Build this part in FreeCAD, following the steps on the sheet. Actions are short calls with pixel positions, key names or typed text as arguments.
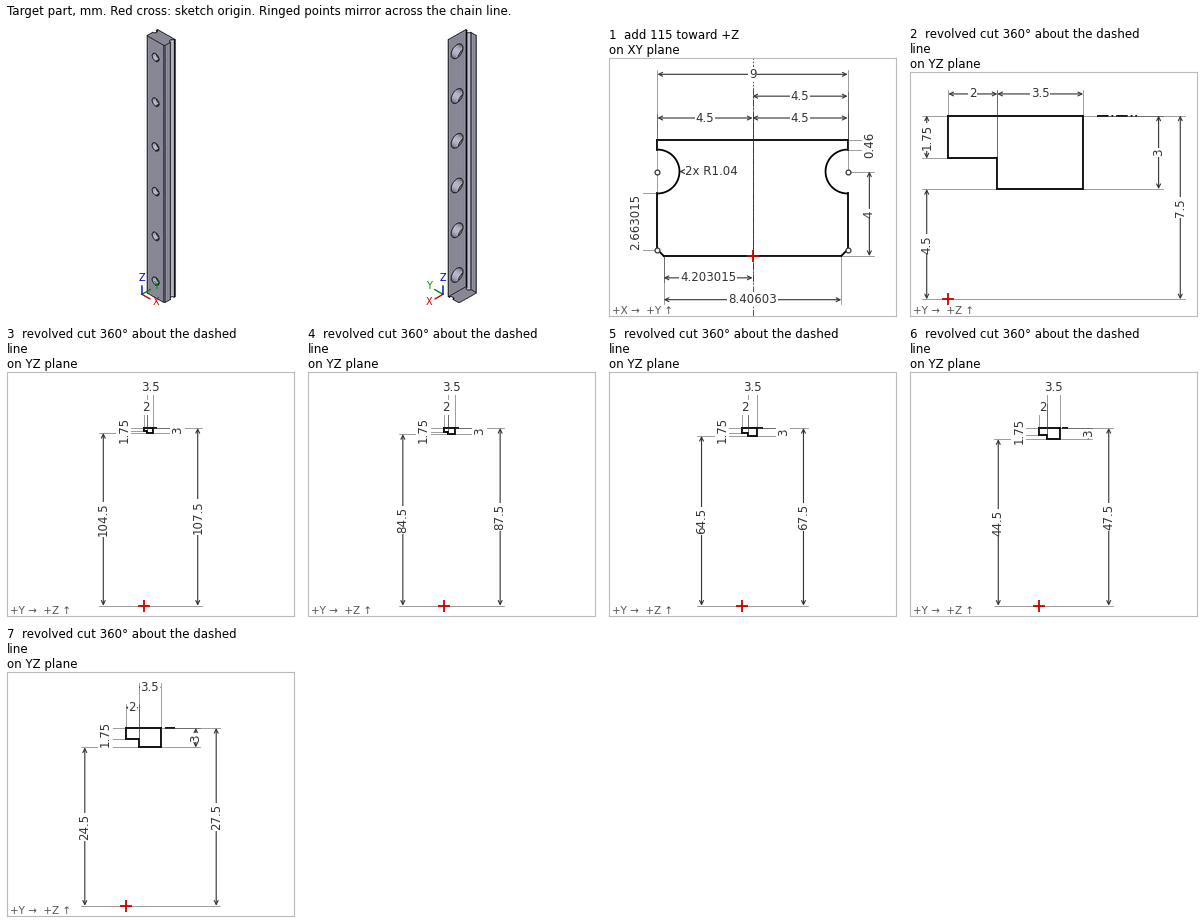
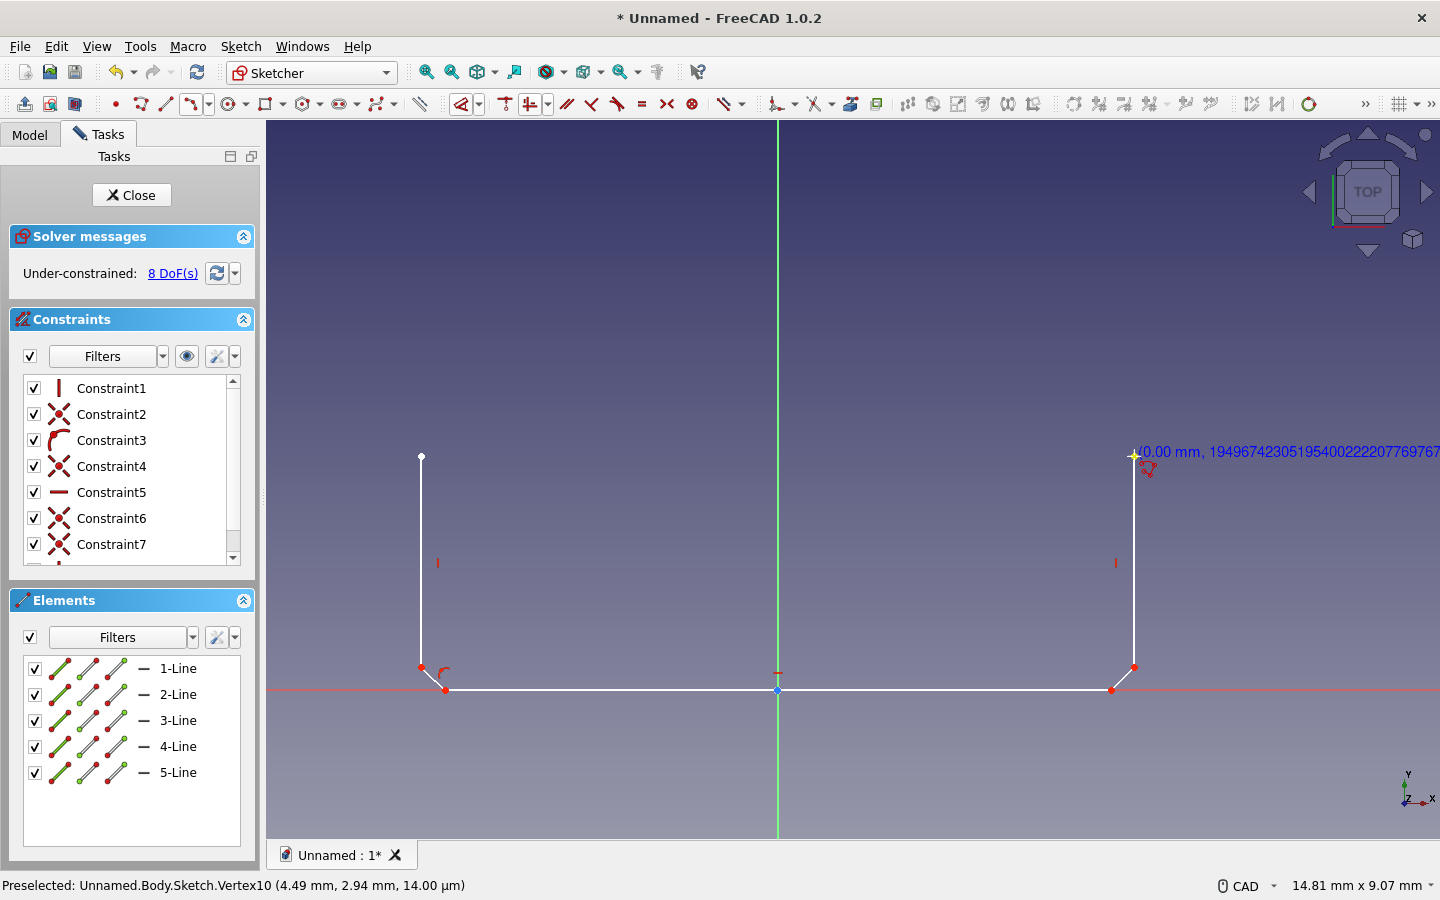
click(1134, 291)
click(1134, 254)
click(421, 254)
click(421, 291)
right_click(421, 291)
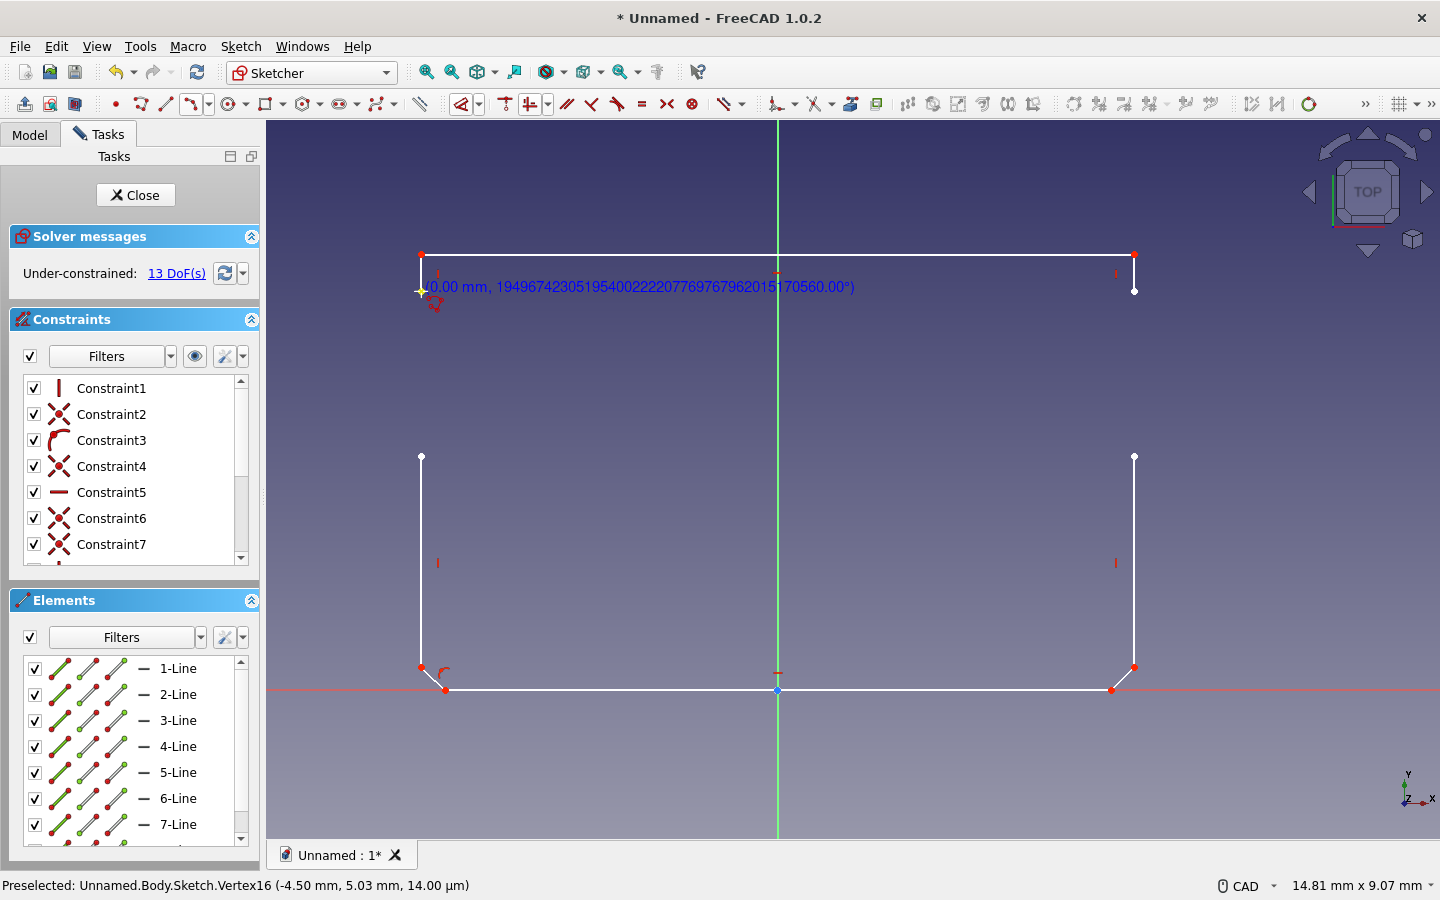
click(190, 104)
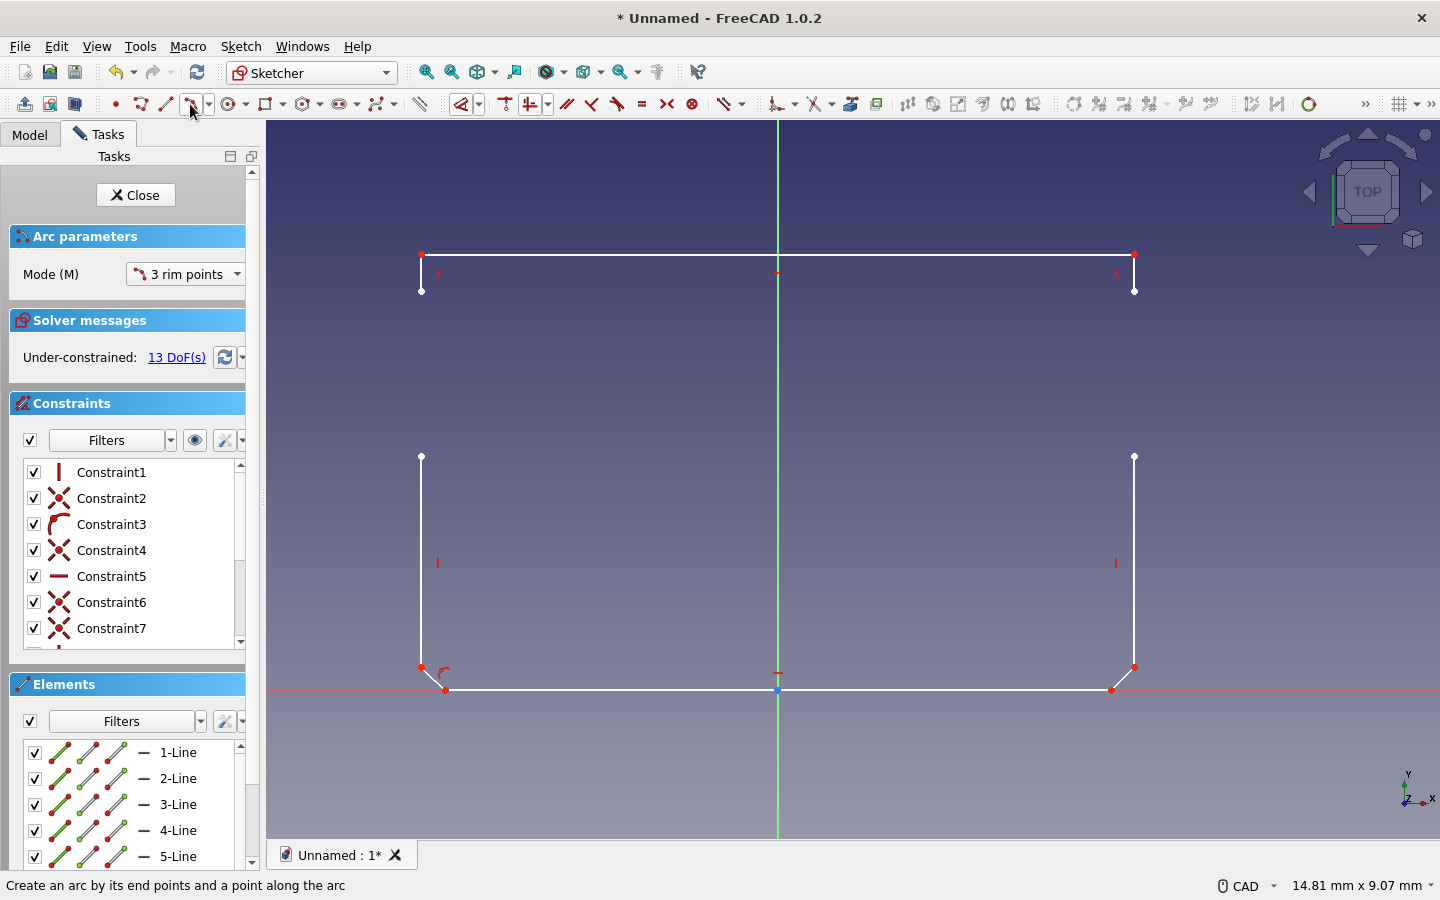
click(1134, 457)
click(1134, 292)
click(1052, 373)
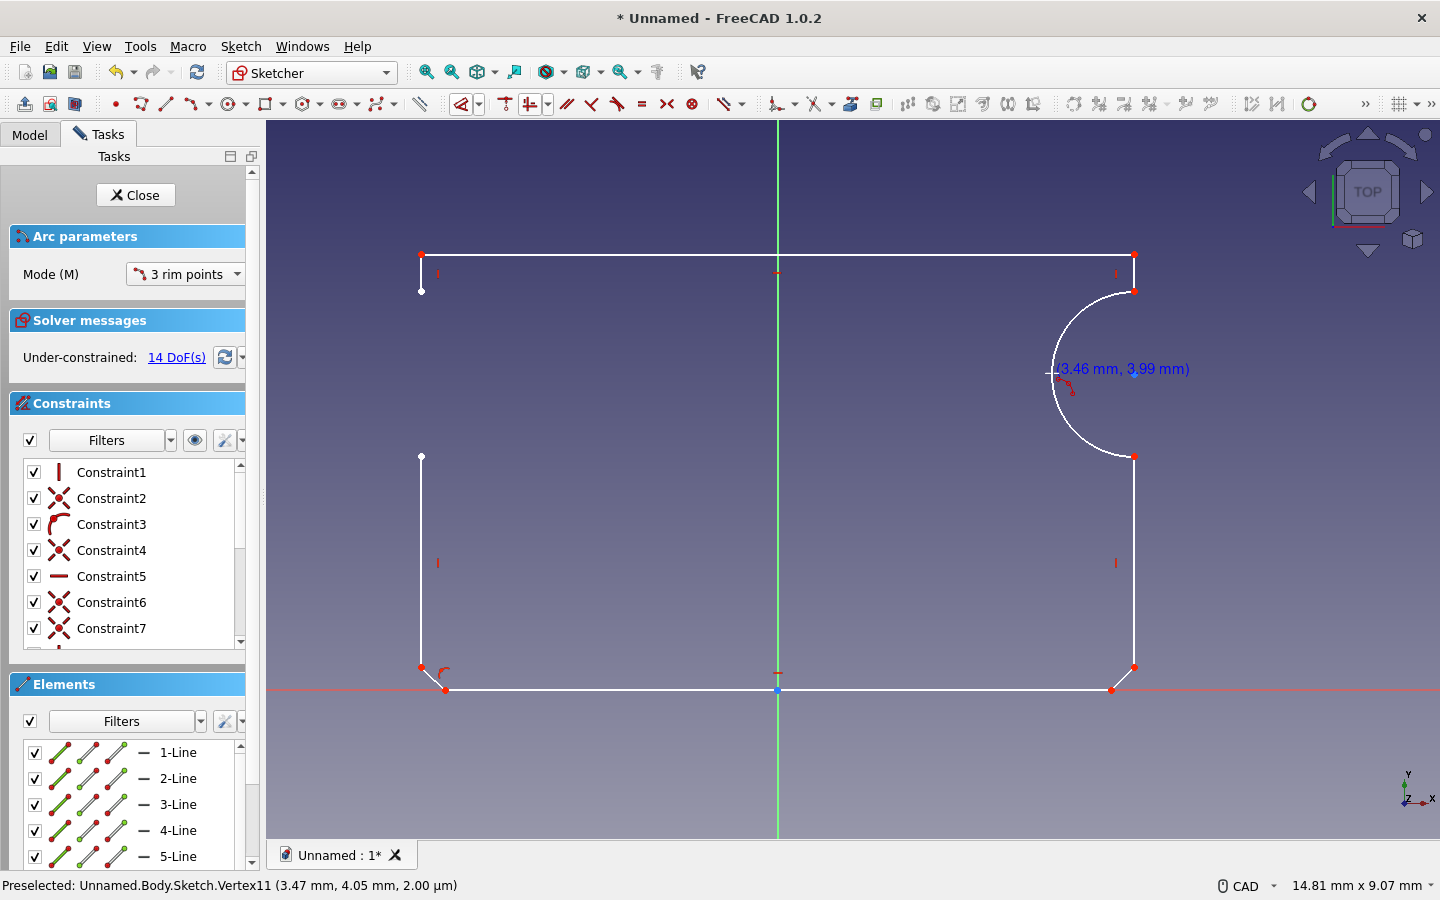
click(421, 292)
click(421, 457)
click(504, 373)
key(Escape)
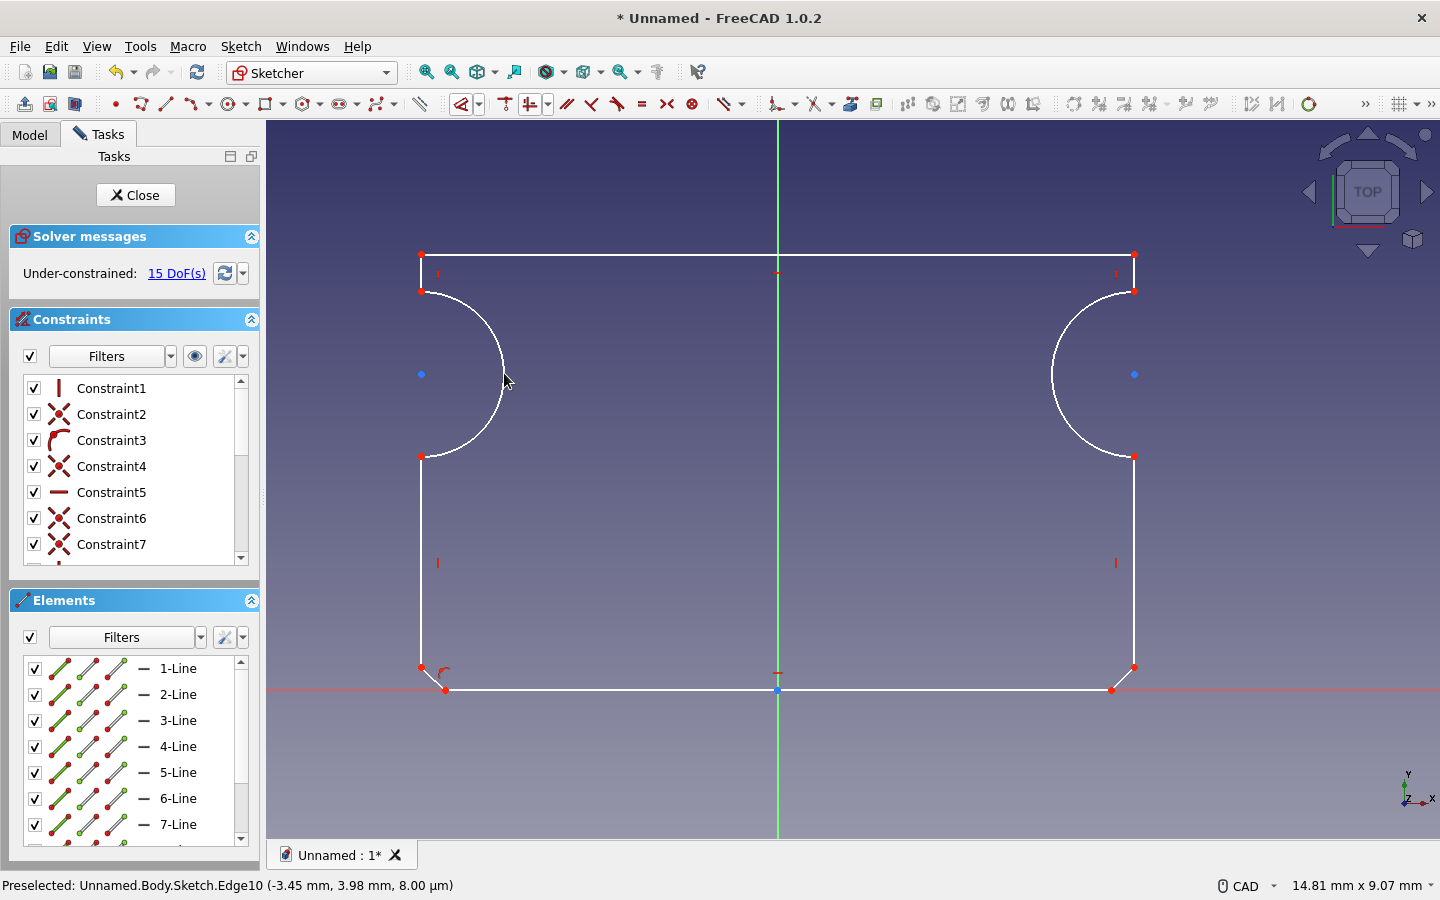
click(1068, 326)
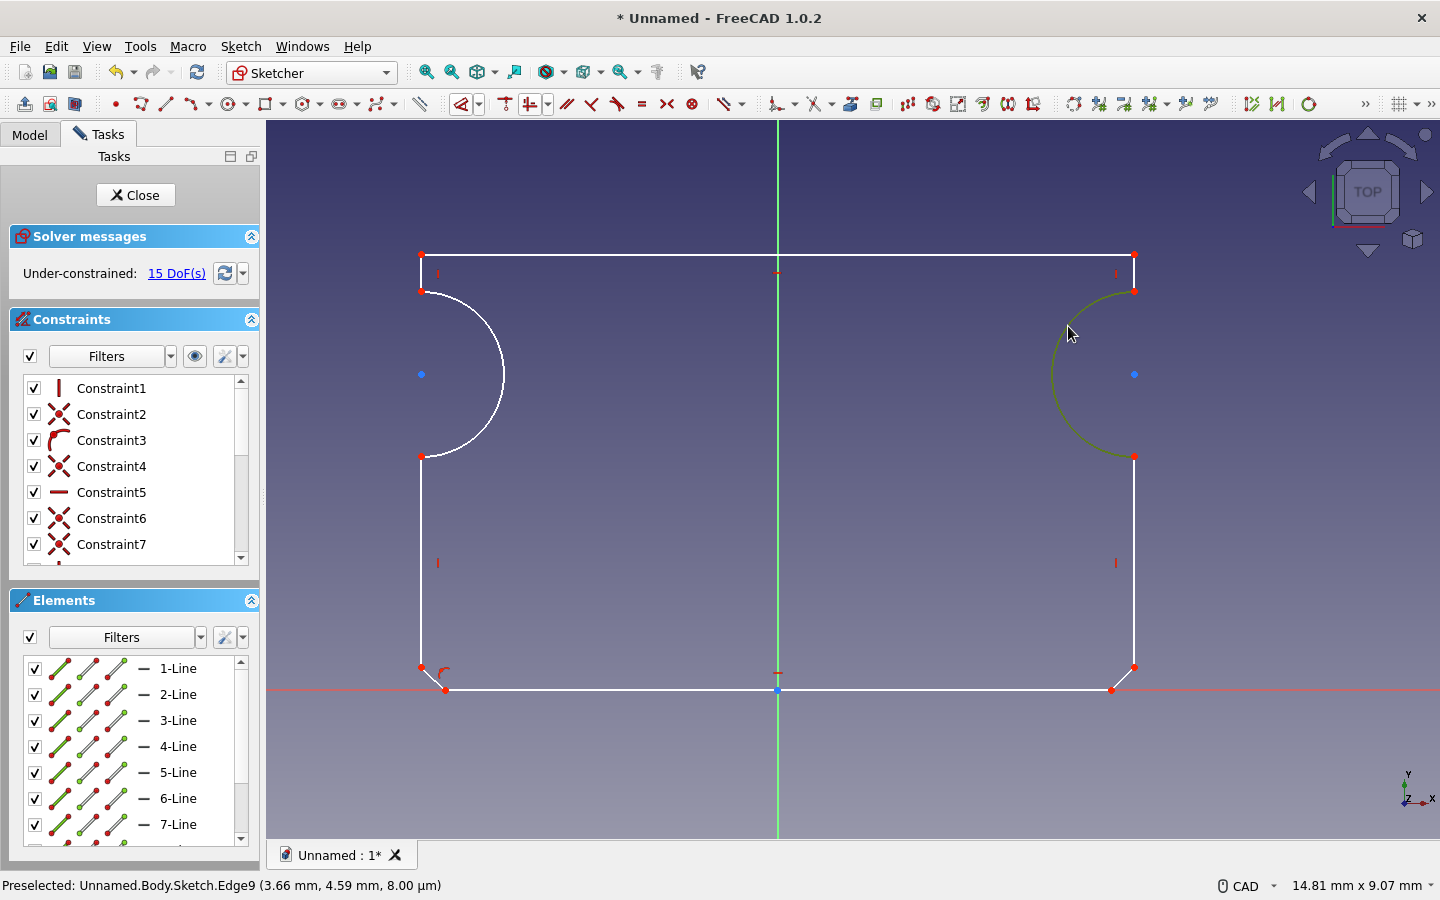
click(488, 423)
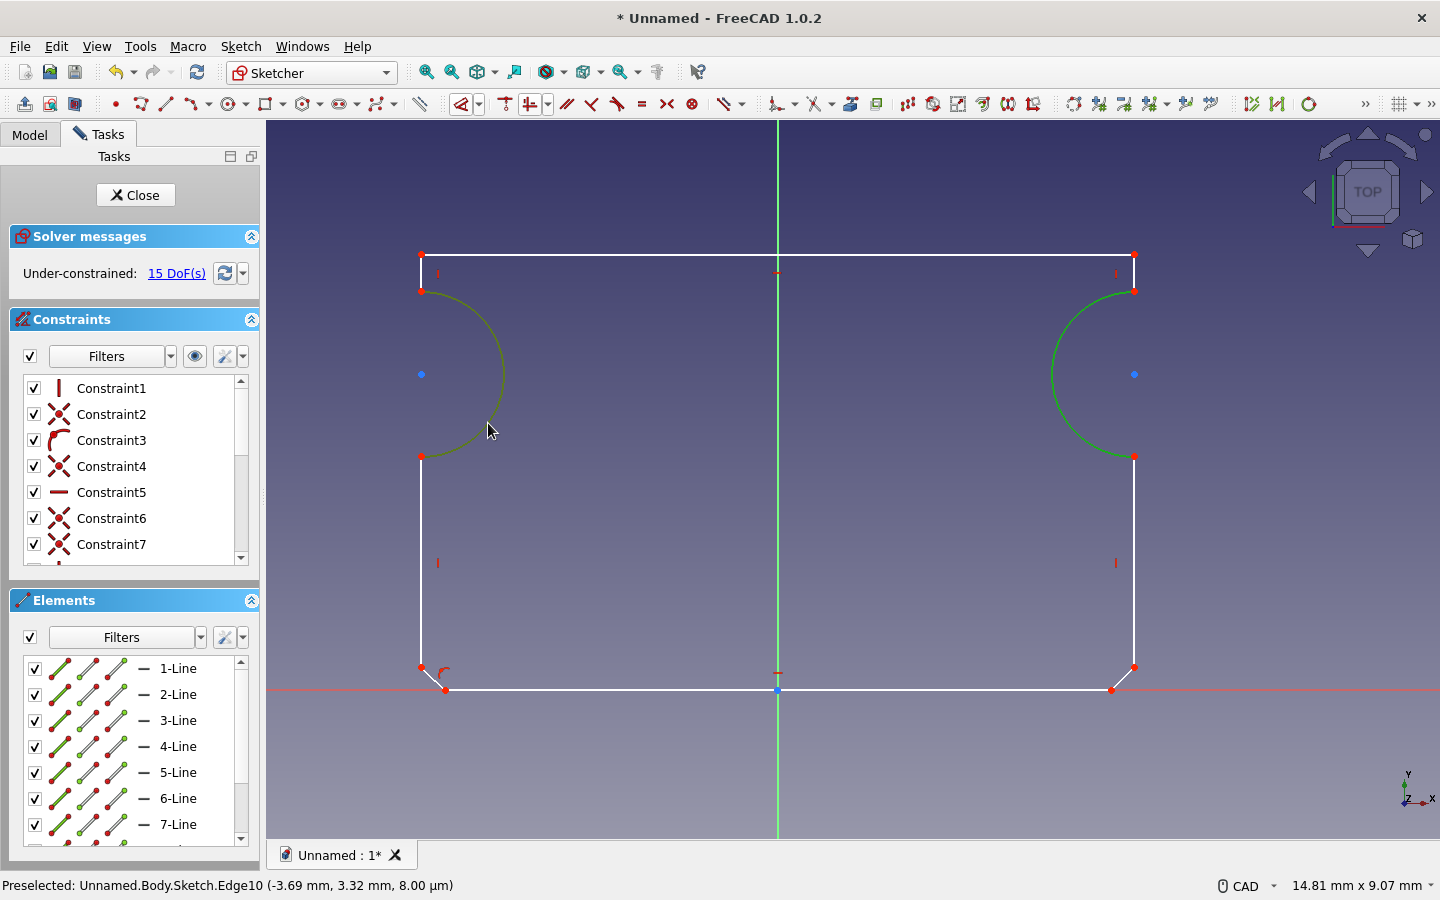
key(e)